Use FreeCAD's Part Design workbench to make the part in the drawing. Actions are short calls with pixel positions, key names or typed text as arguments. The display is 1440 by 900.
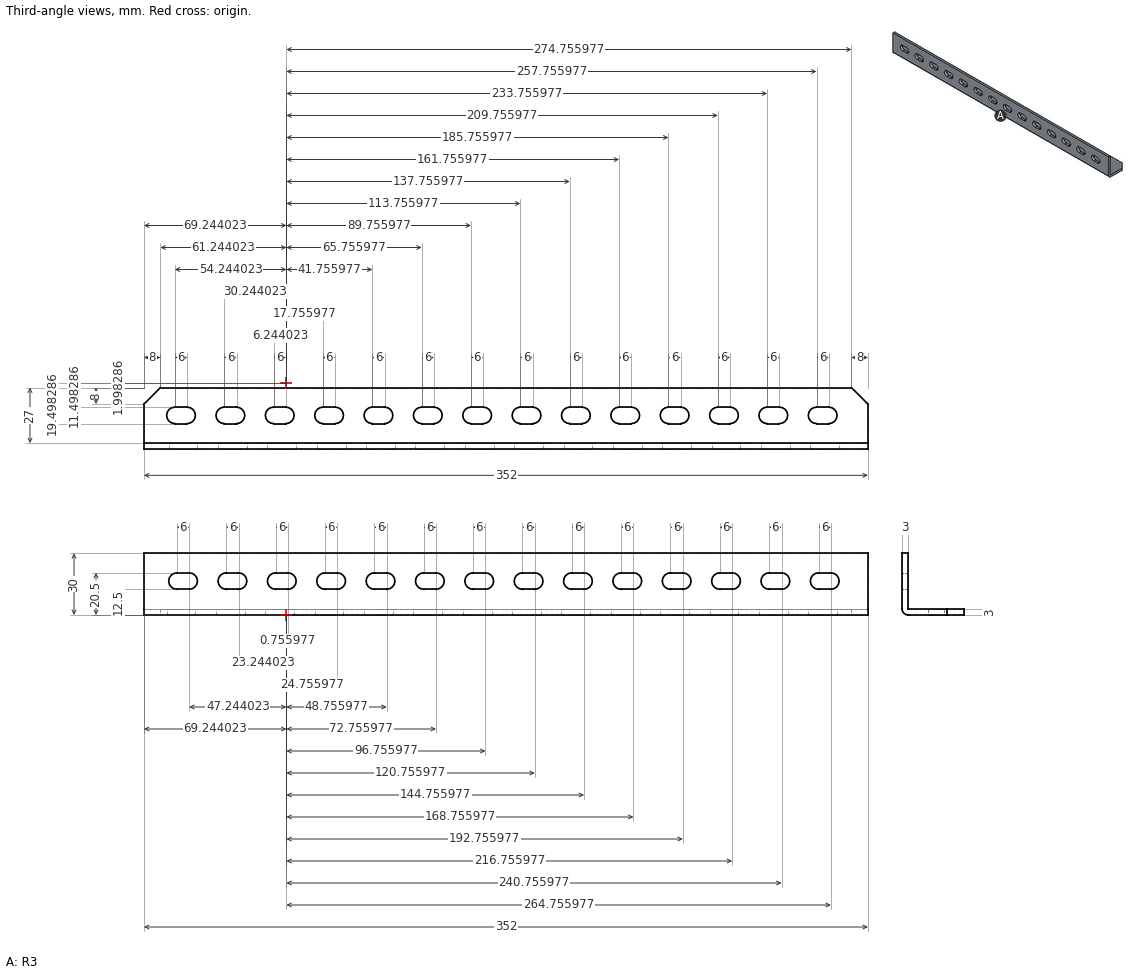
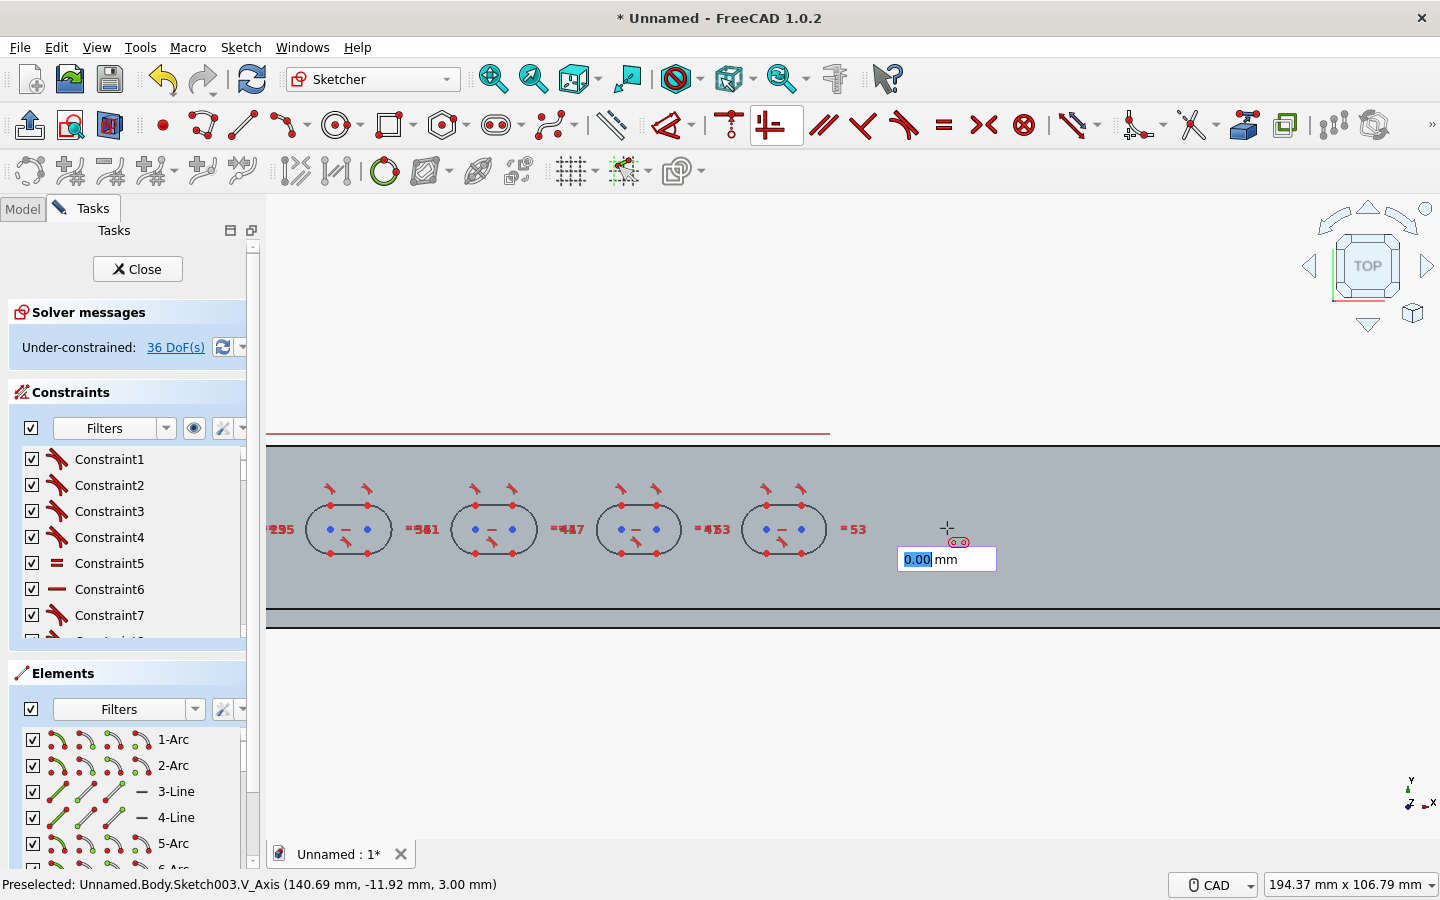
click(929, 504)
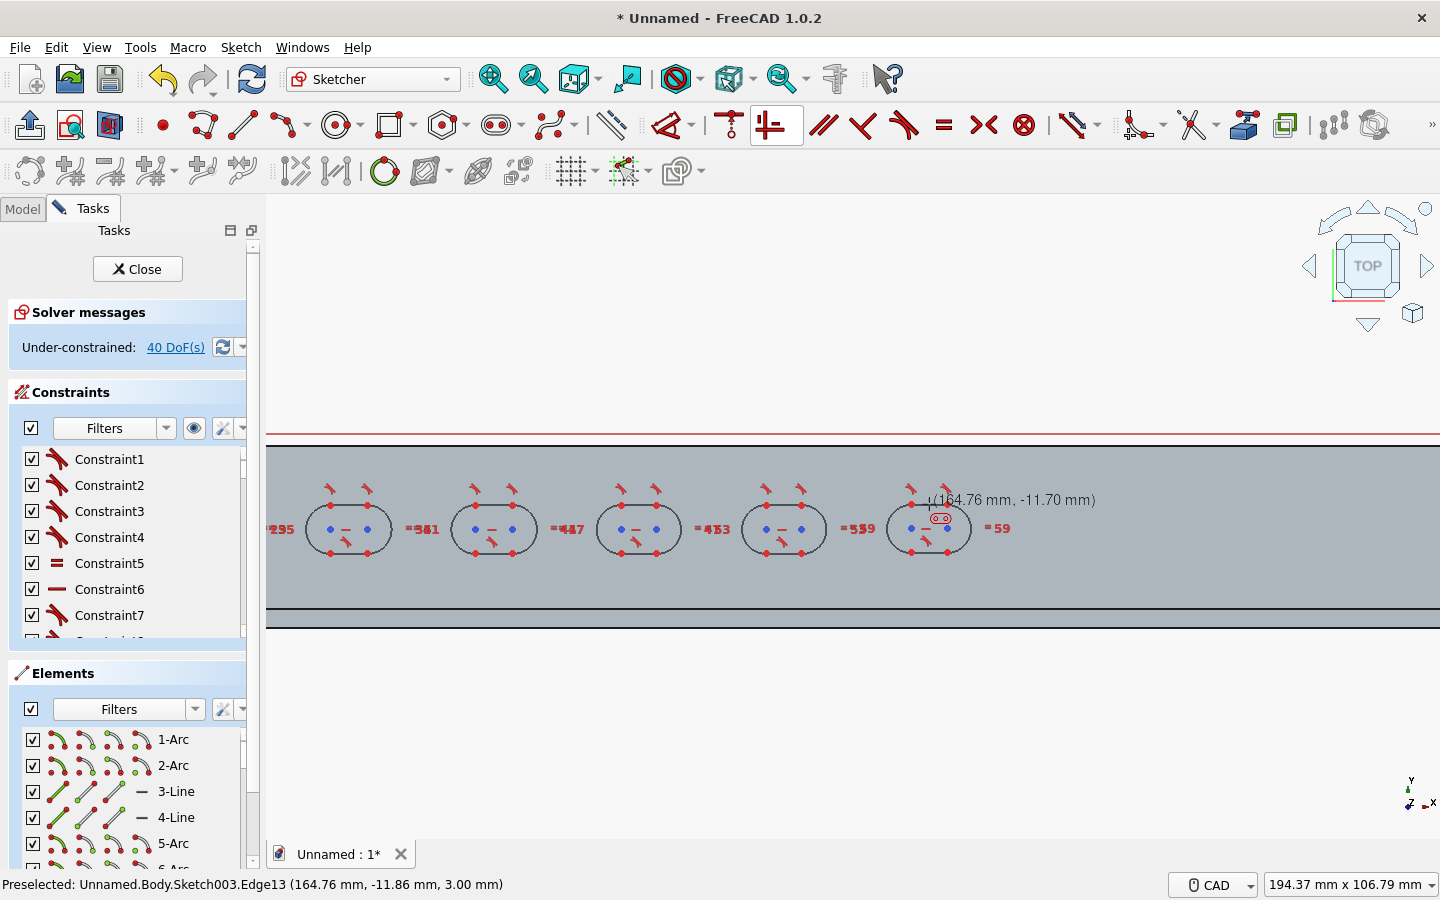
click(1056, 528)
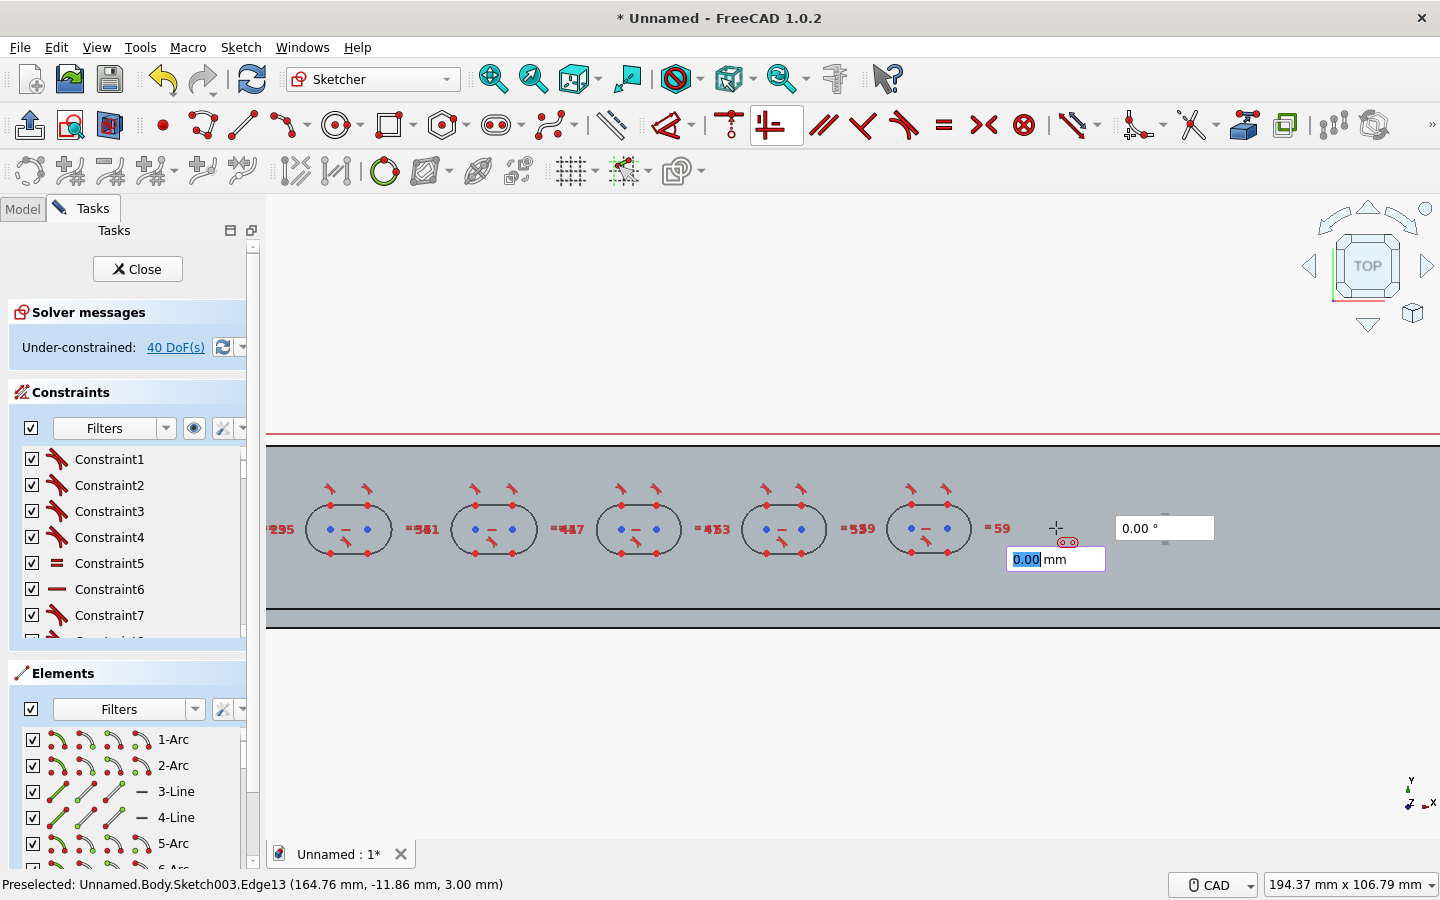
click(1092, 528)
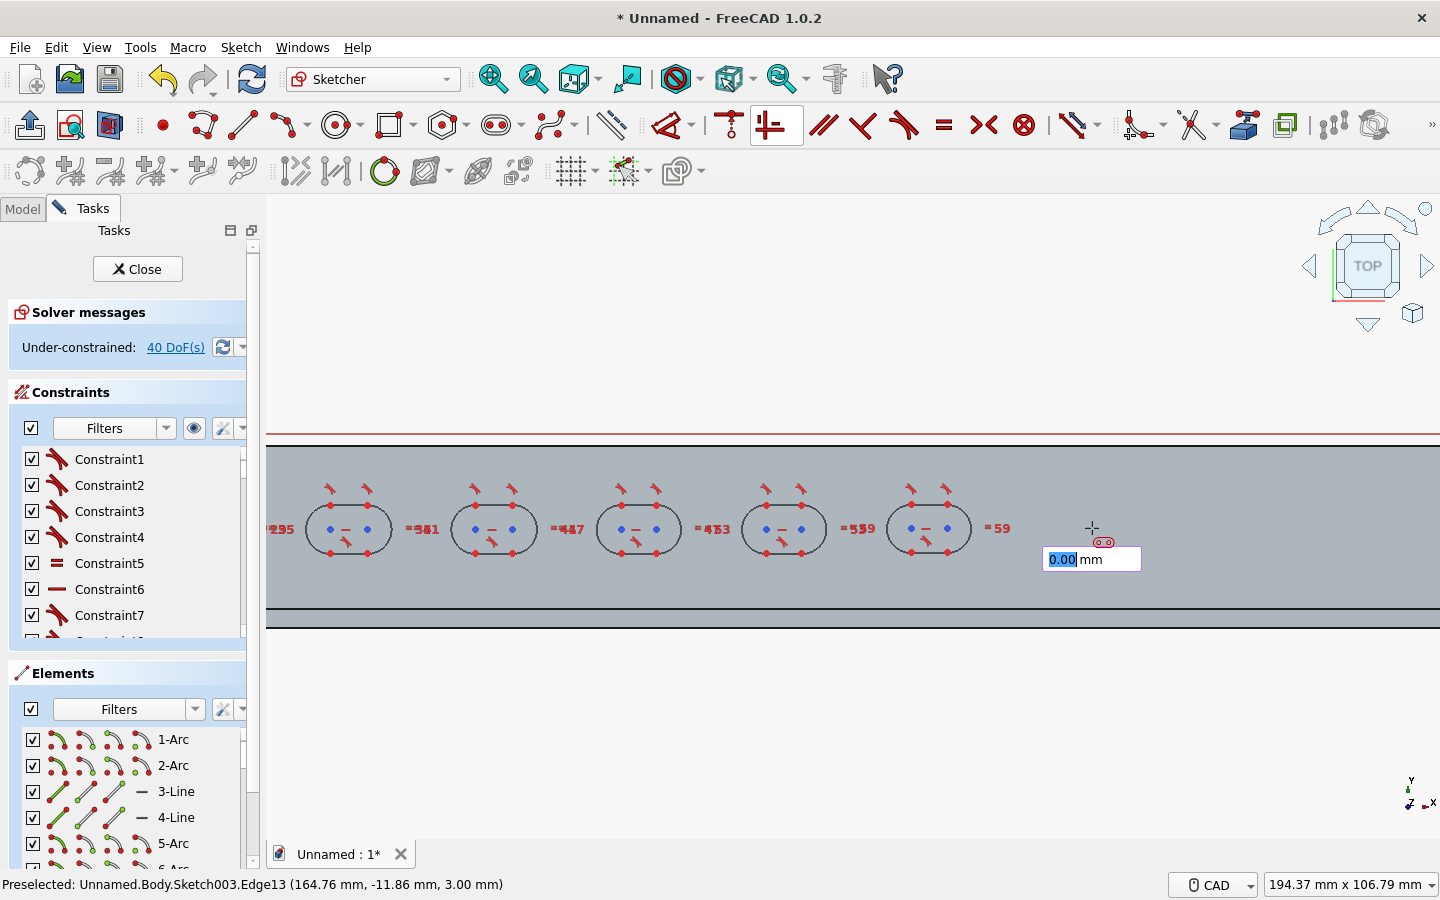
click(1074, 504)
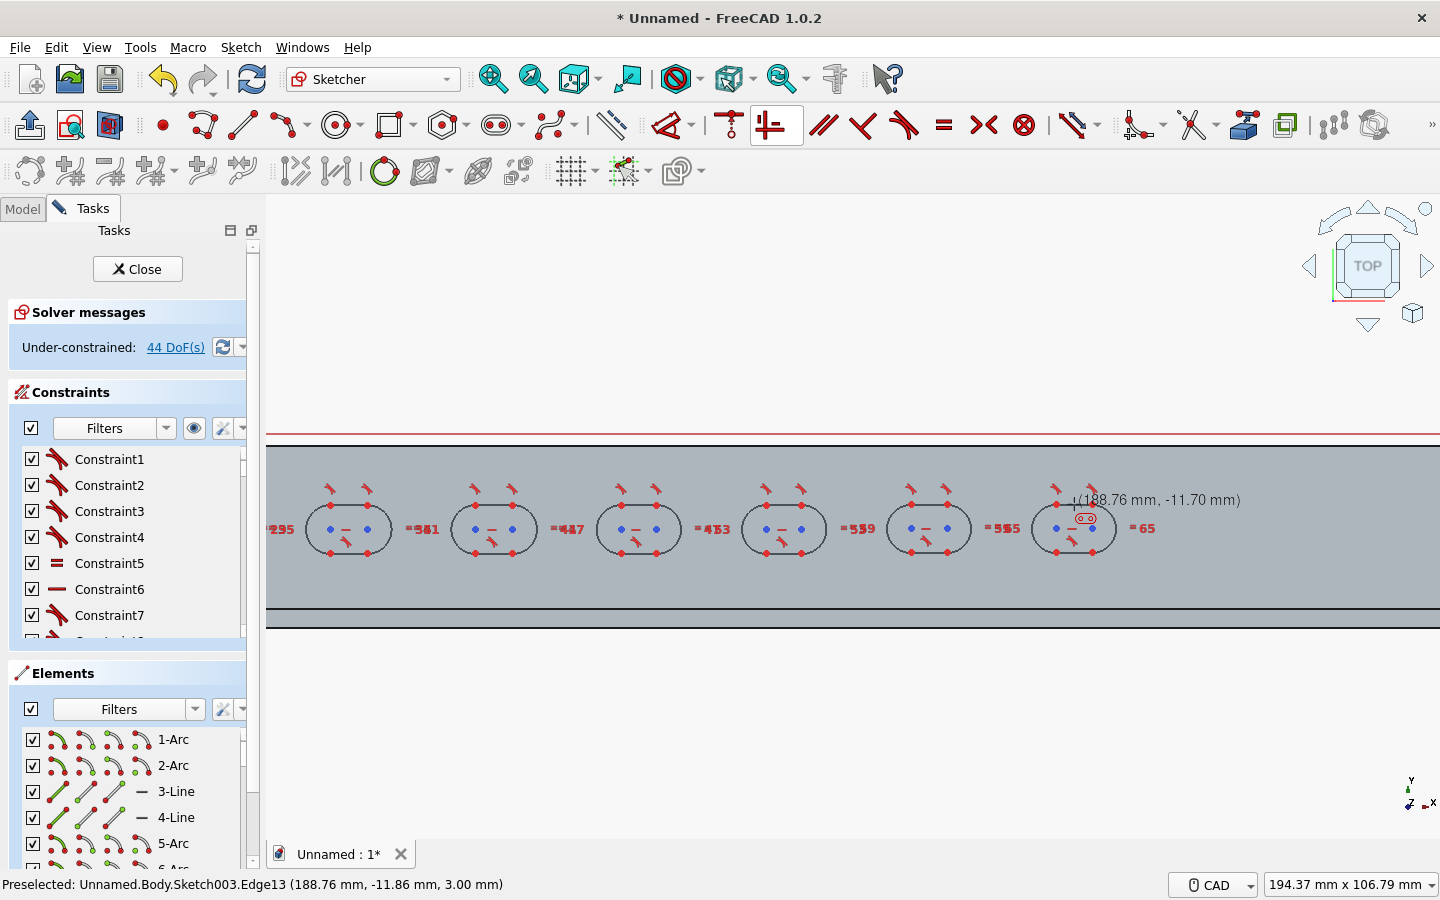
click(1201, 528)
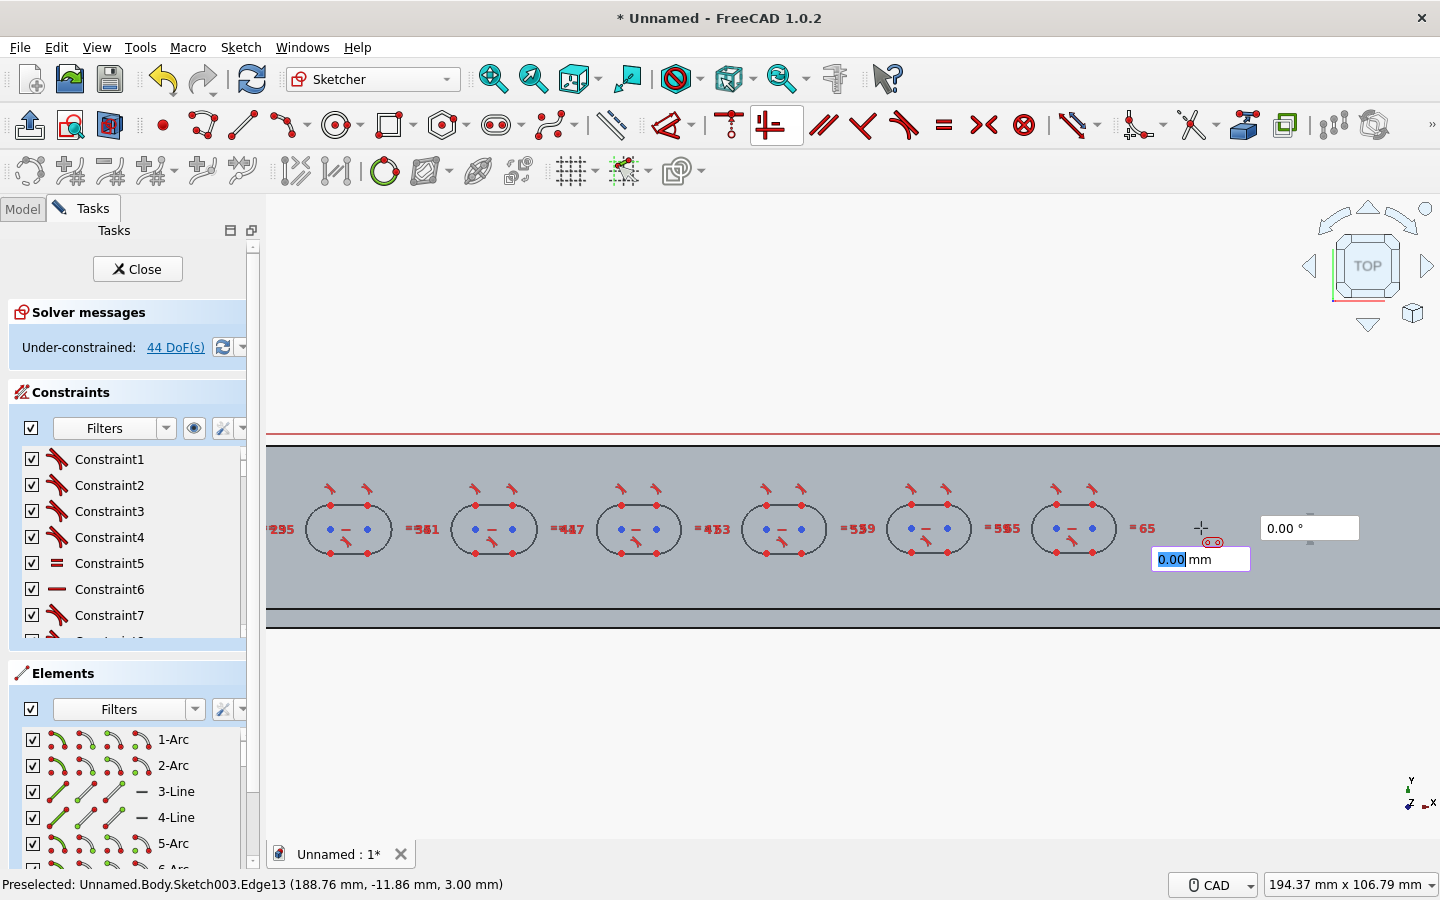
click(1237, 528)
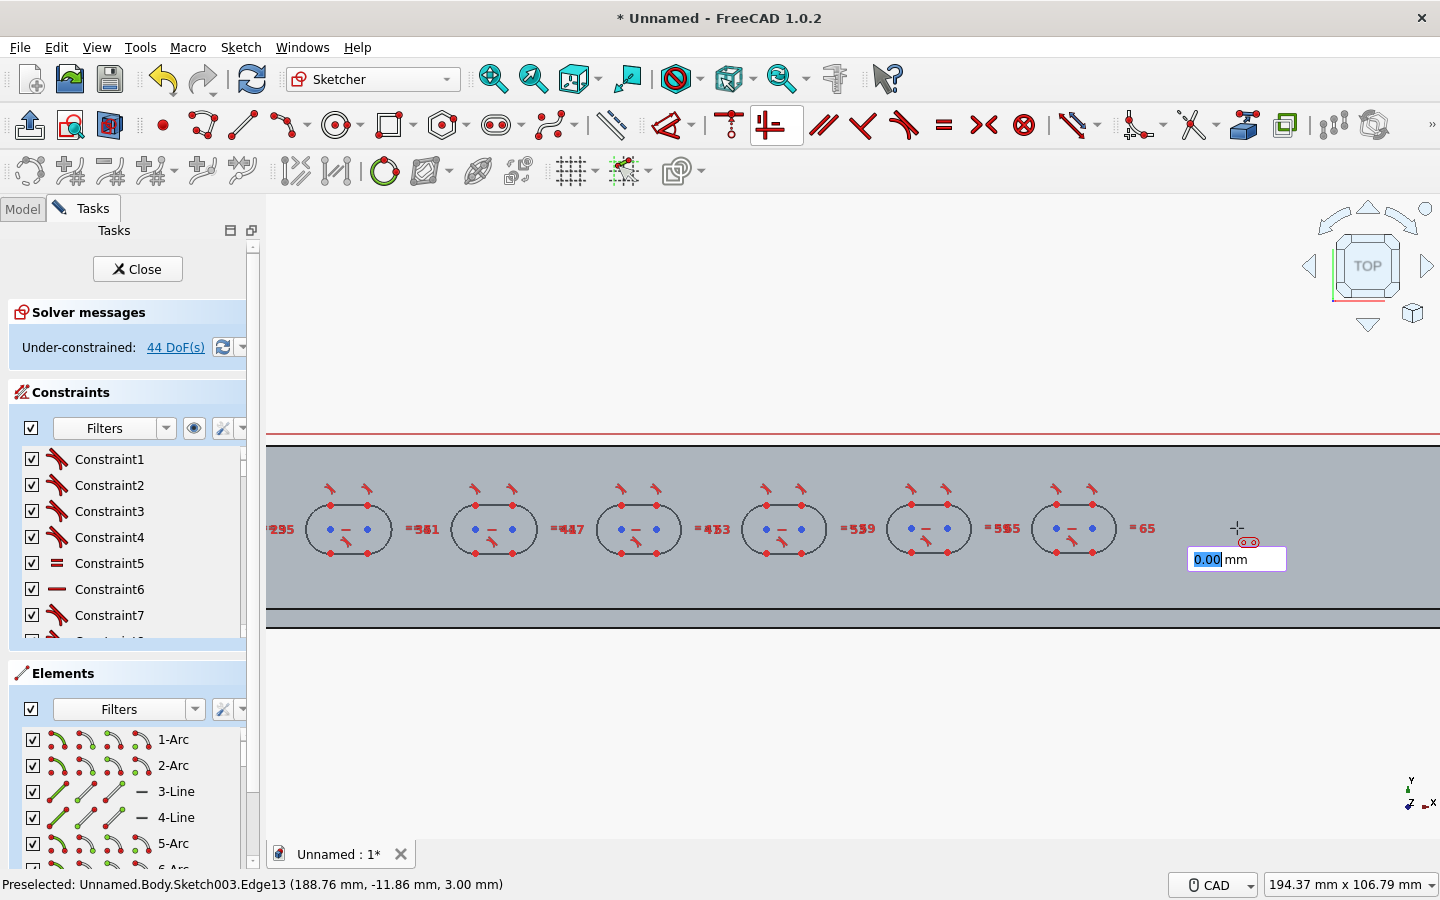
click(1219, 504)